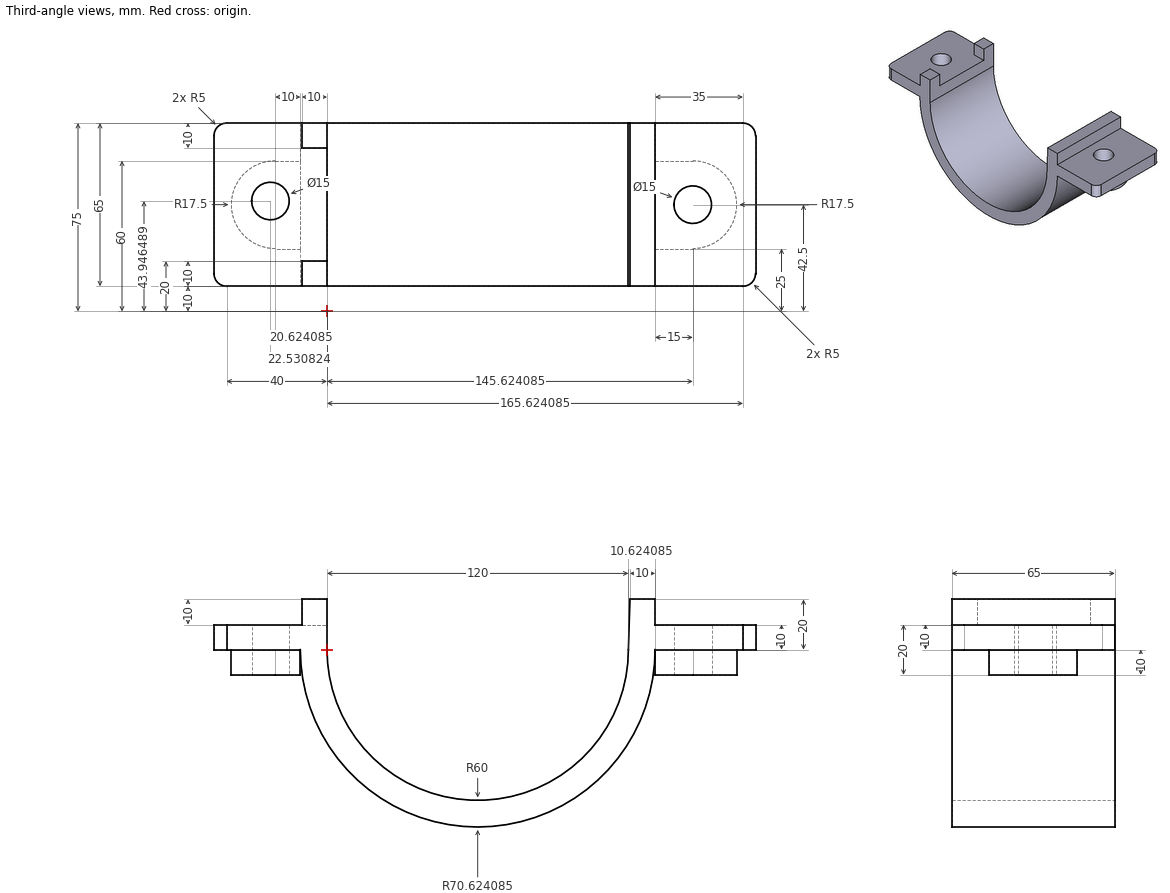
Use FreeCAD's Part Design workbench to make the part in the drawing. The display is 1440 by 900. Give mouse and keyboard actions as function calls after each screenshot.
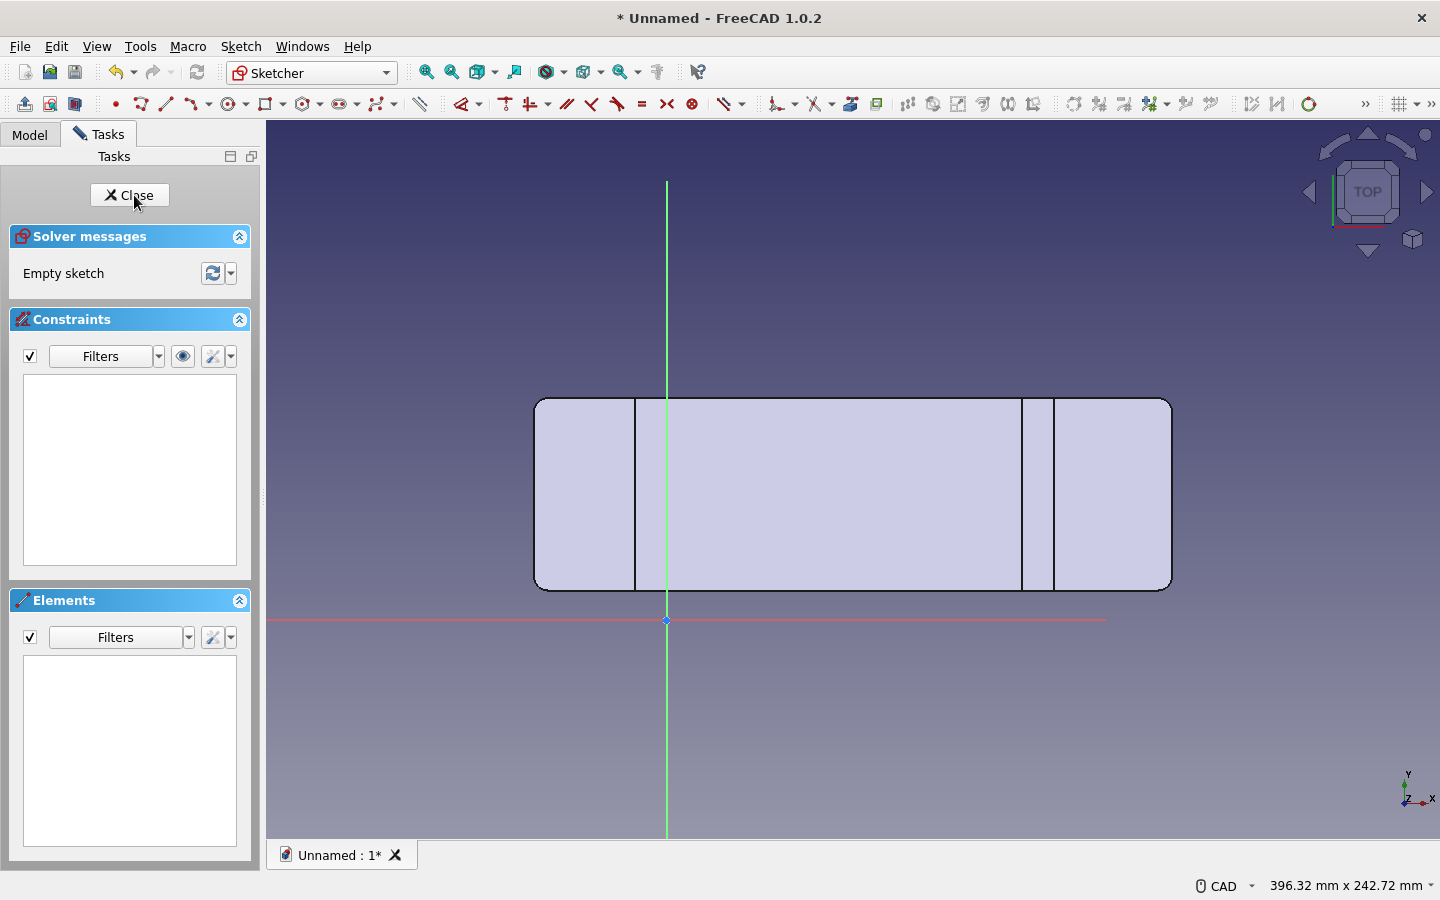
scroll(1182, 498, up, 8)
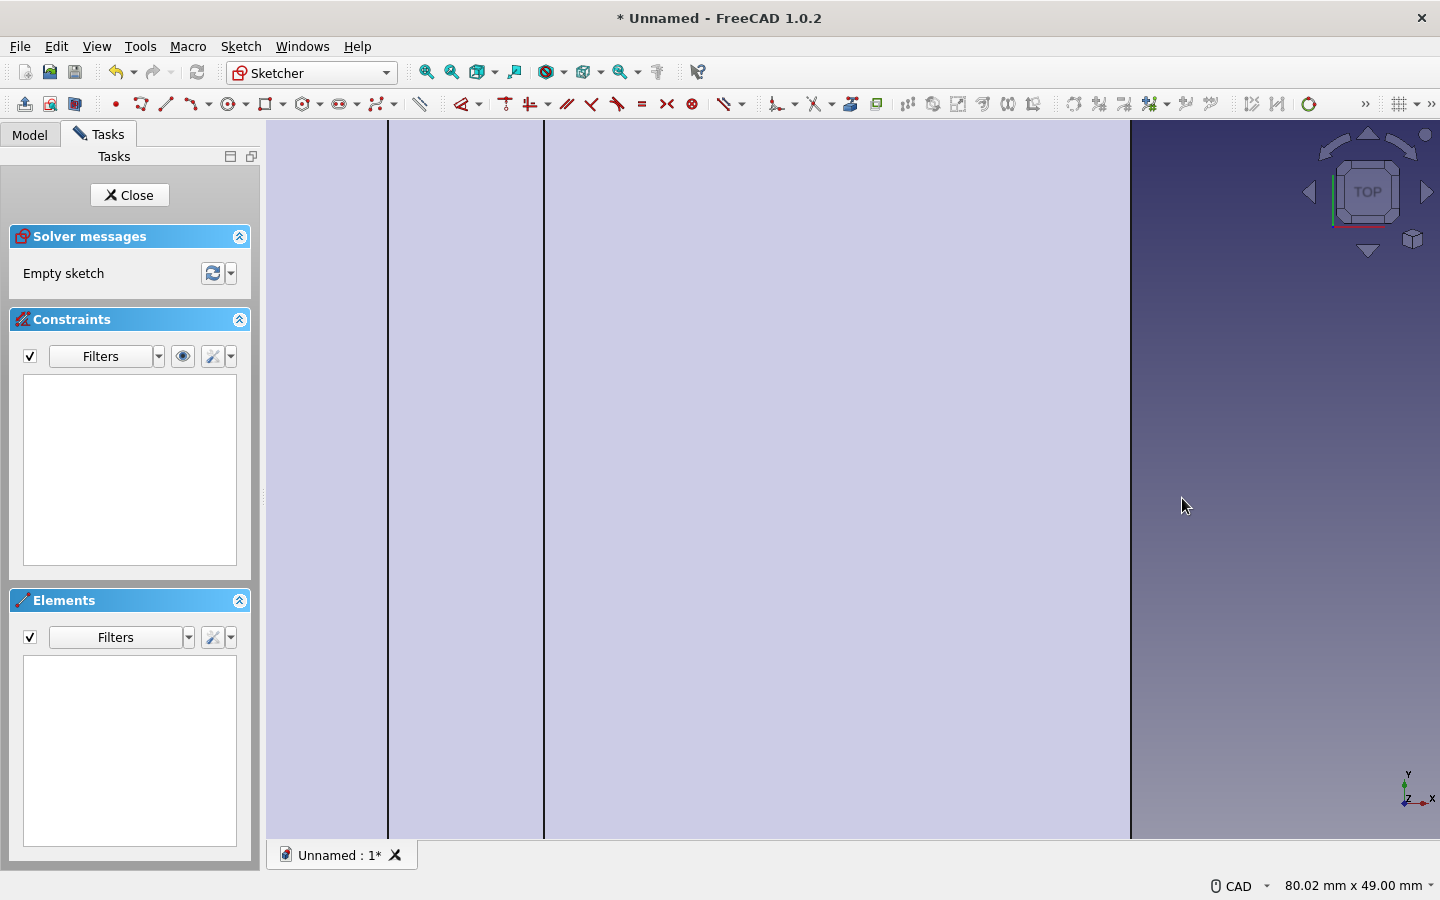
key(g)
key(m)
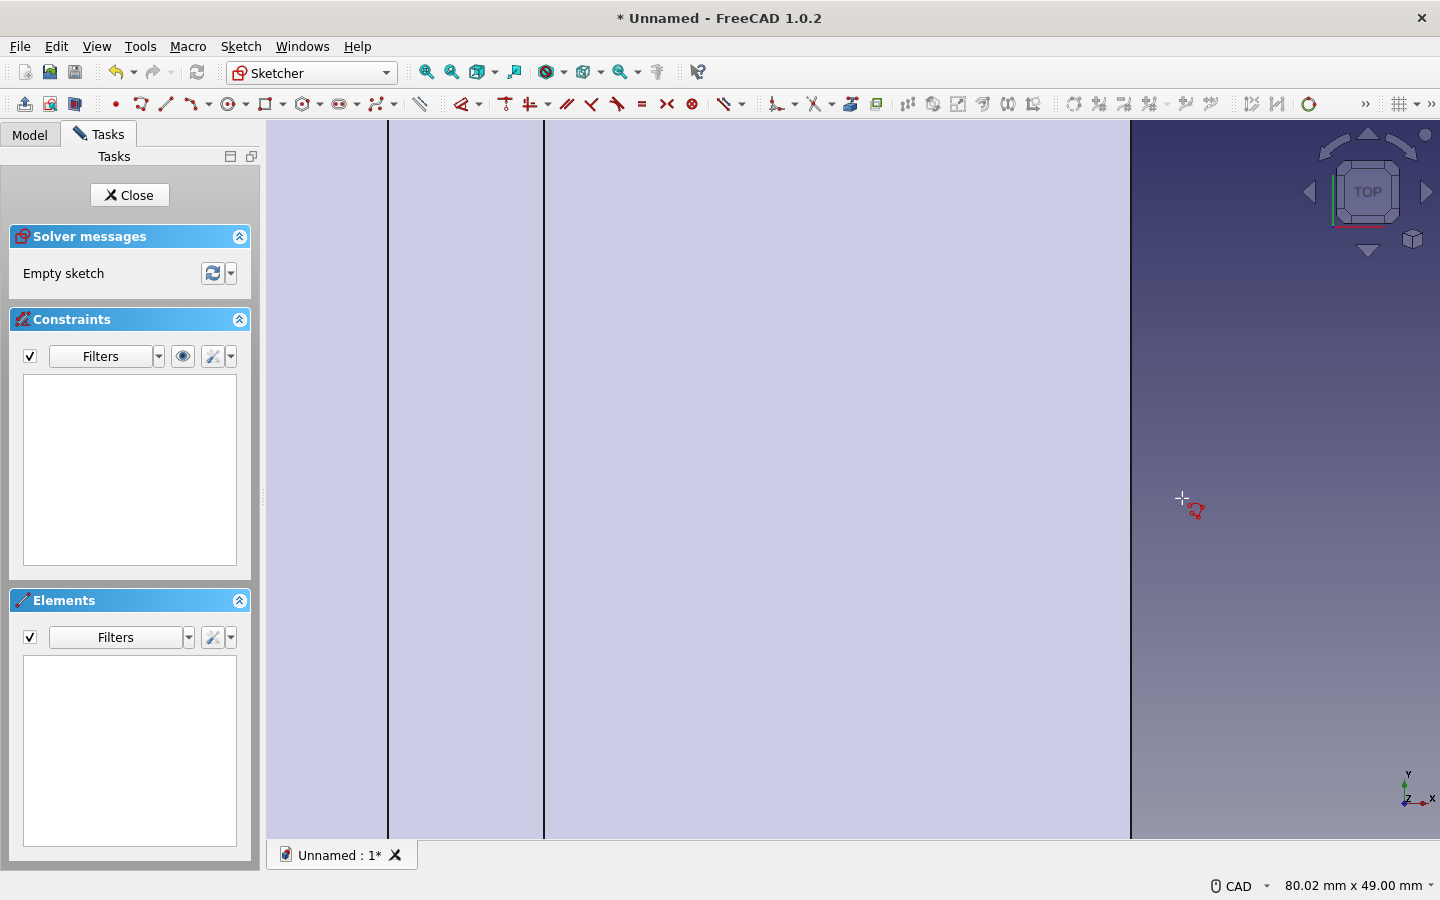
click(764, 734)
click(544, 734)
click(544, 221)
click(764, 221)
right_click(764, 221)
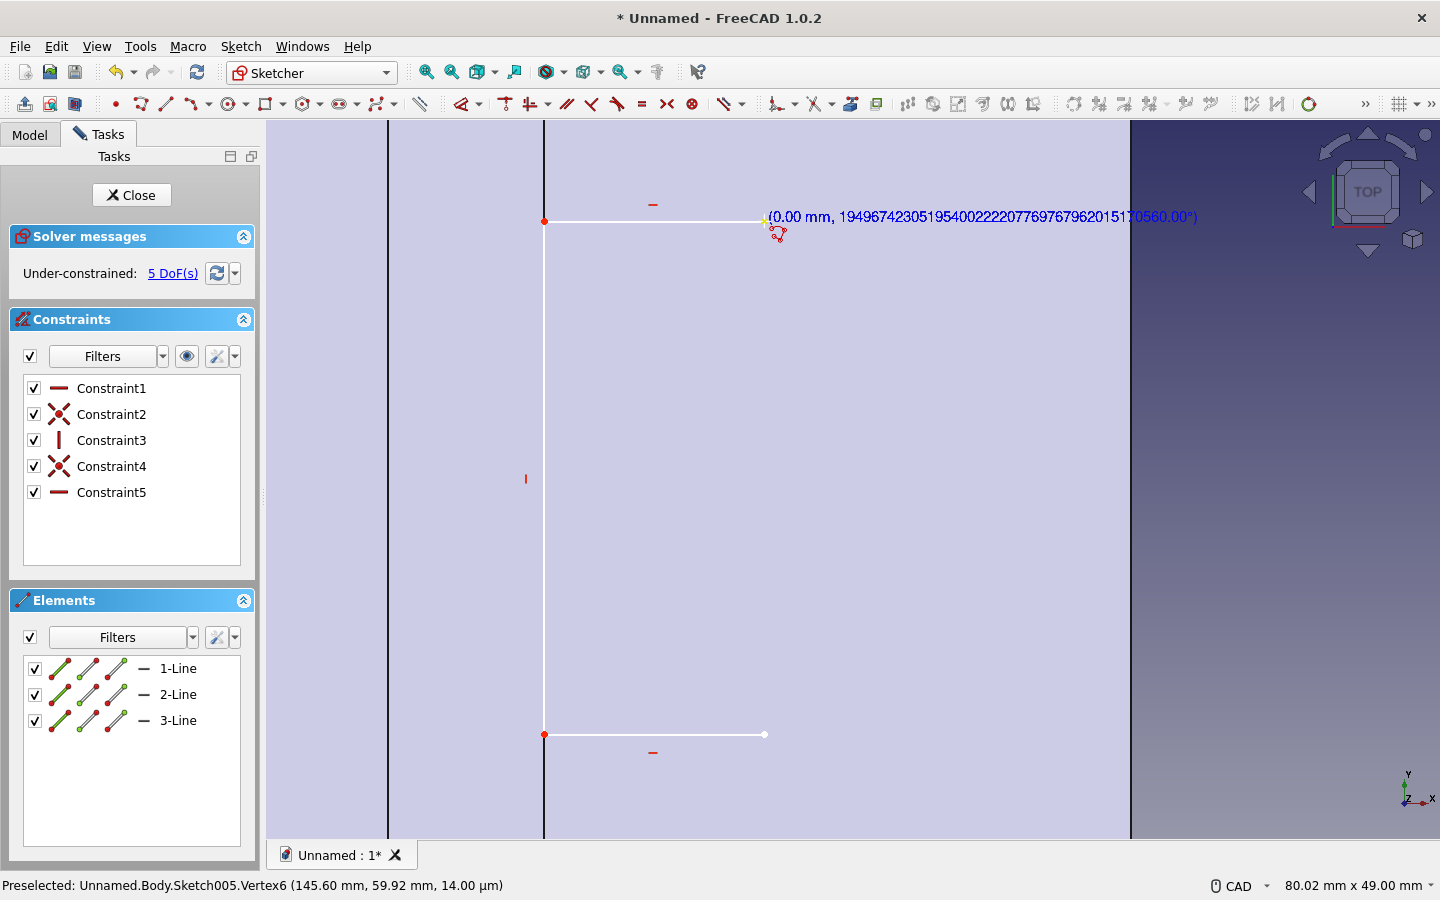
key(g)
key(3)
key(a)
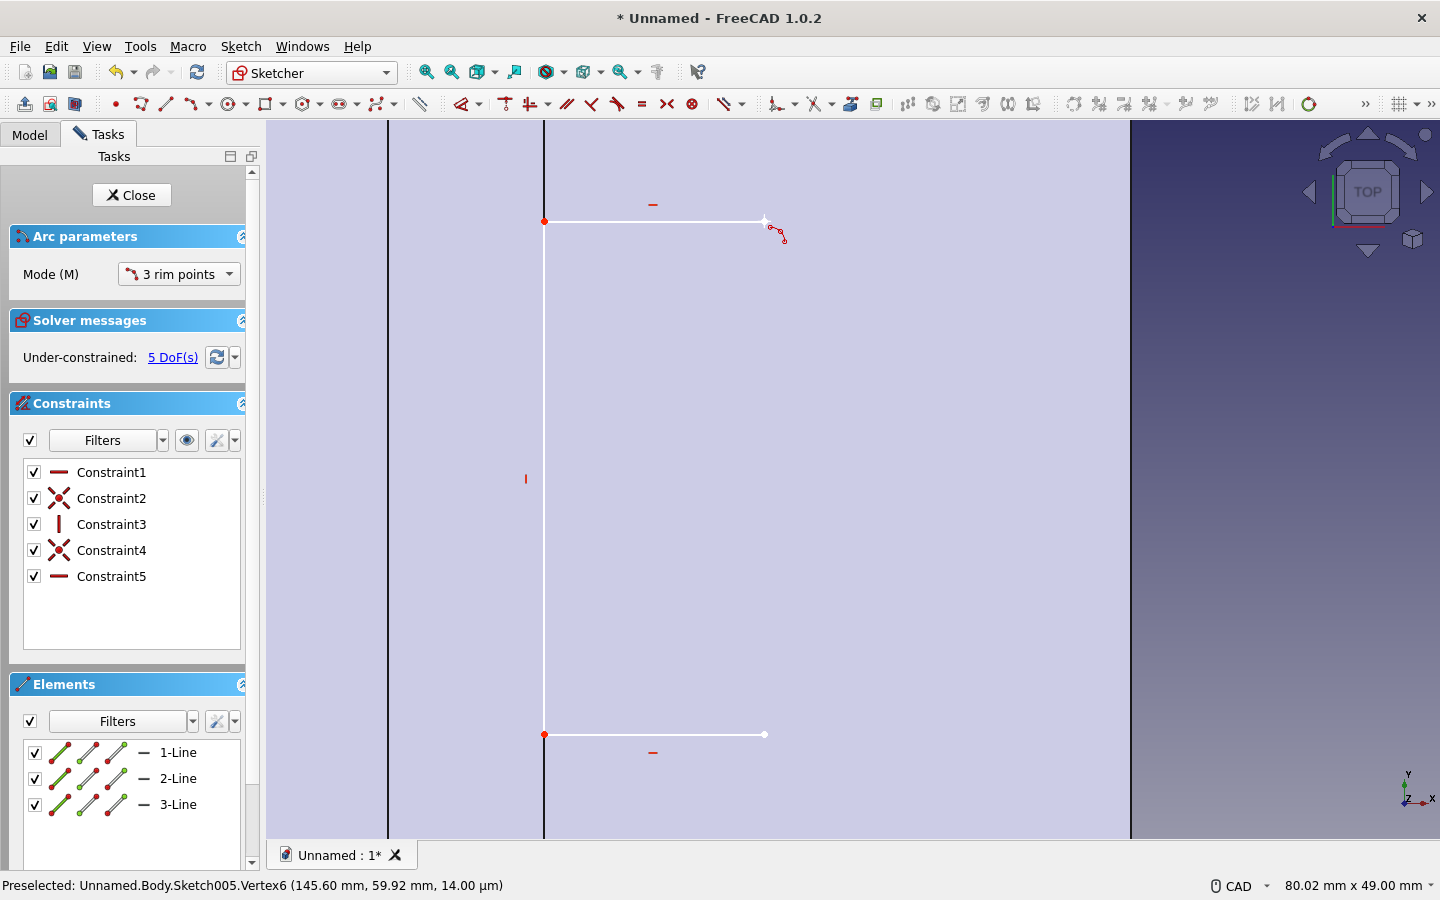
click(764, 222)
click(764, 735)
click(1021, 478)
key(Escape)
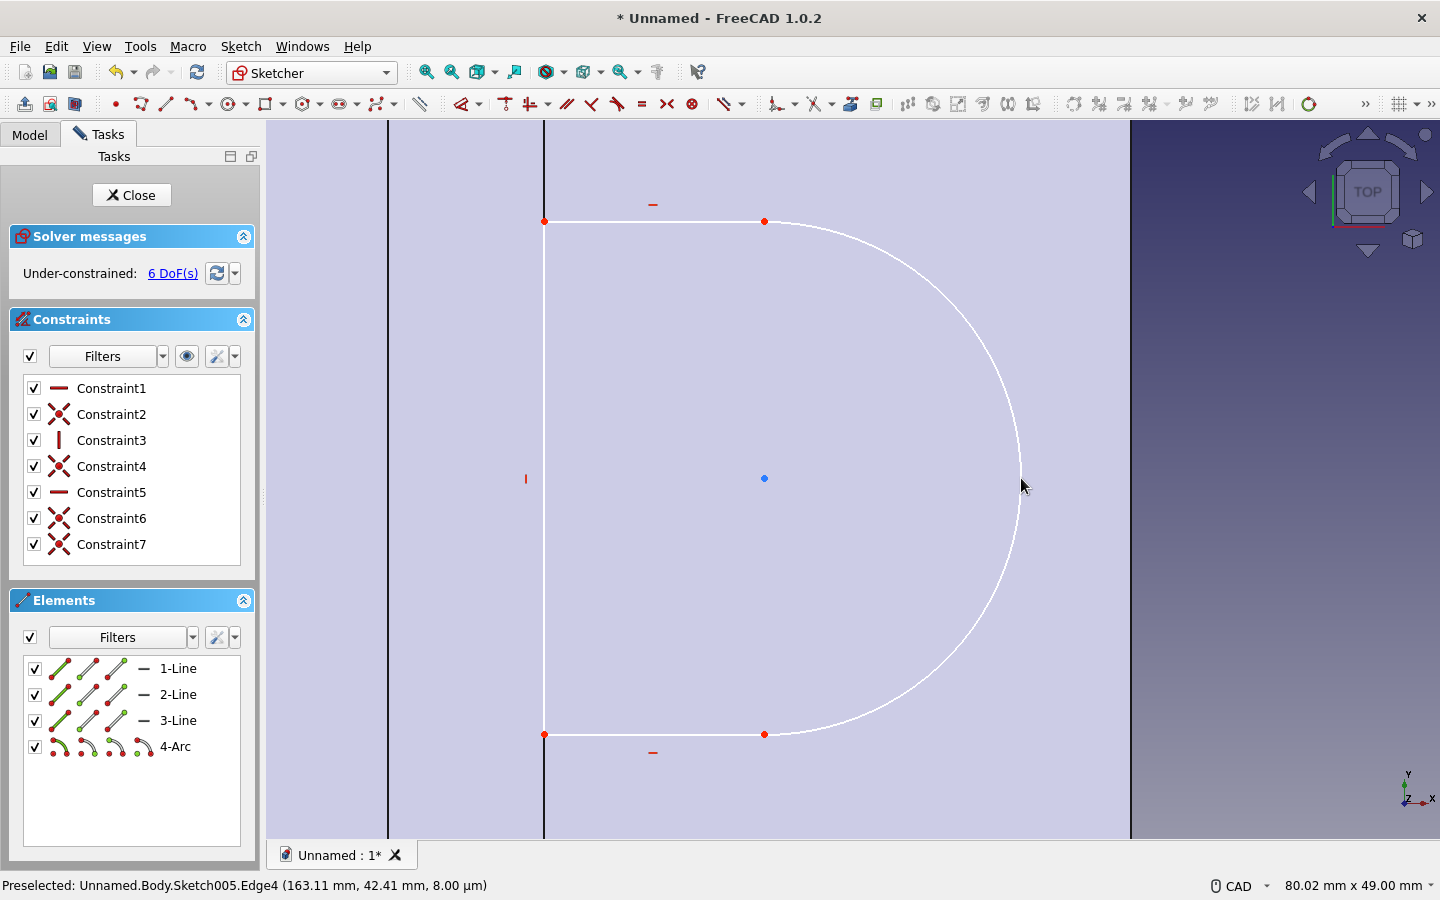
click(698, 735)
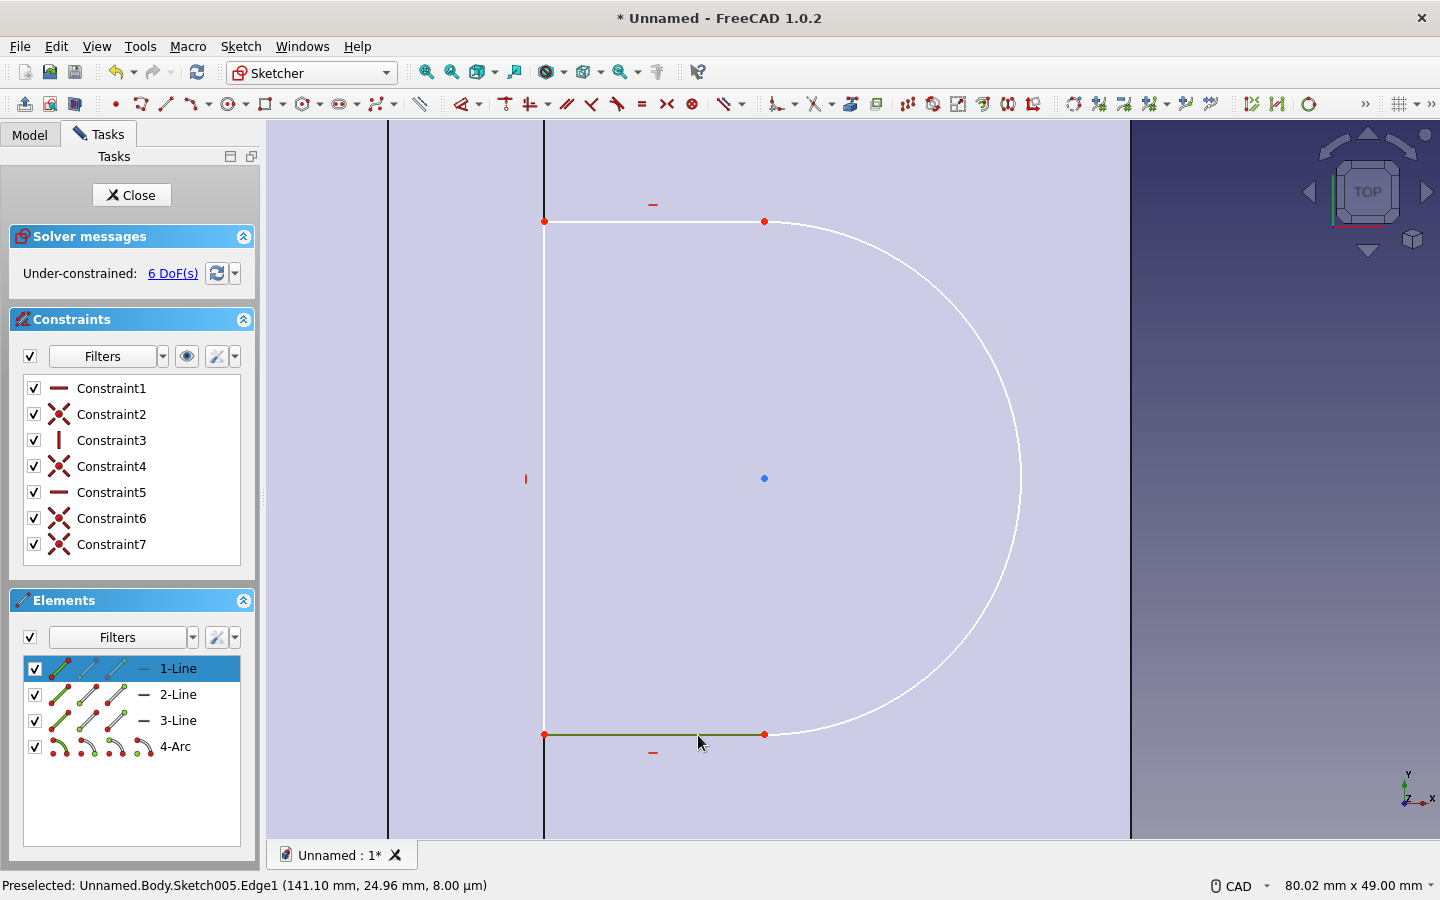
click(972, 629)